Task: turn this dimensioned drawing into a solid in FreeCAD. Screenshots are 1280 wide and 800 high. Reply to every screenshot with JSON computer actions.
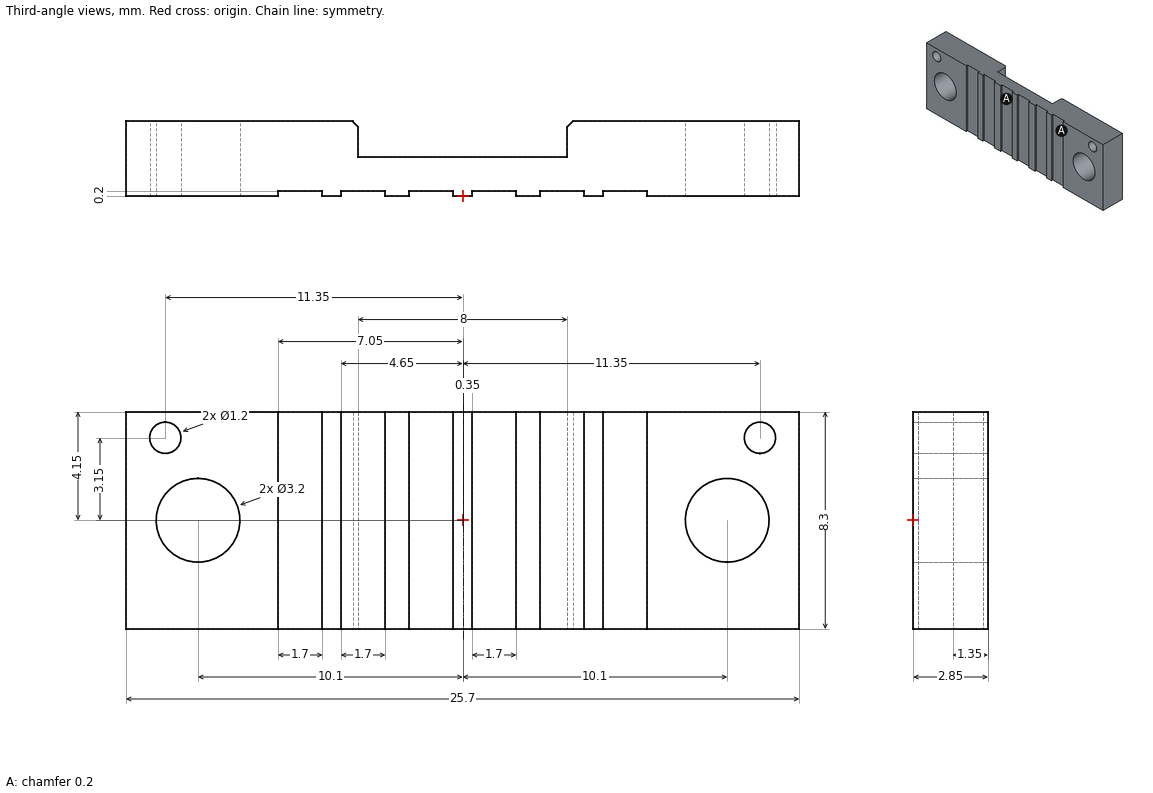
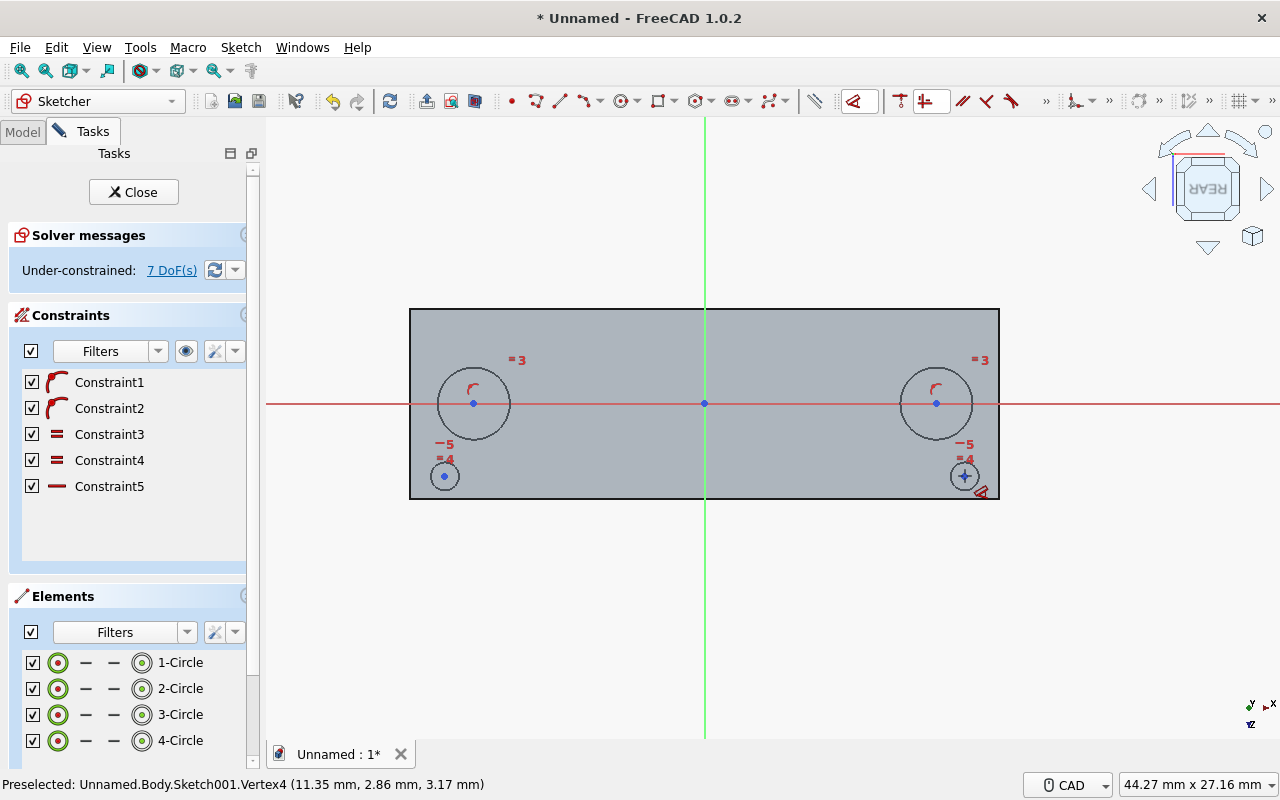
{"action": "left_click", "coordinate": [499, 378]}
{"action": "left_click", "coordinate": [521, 355]}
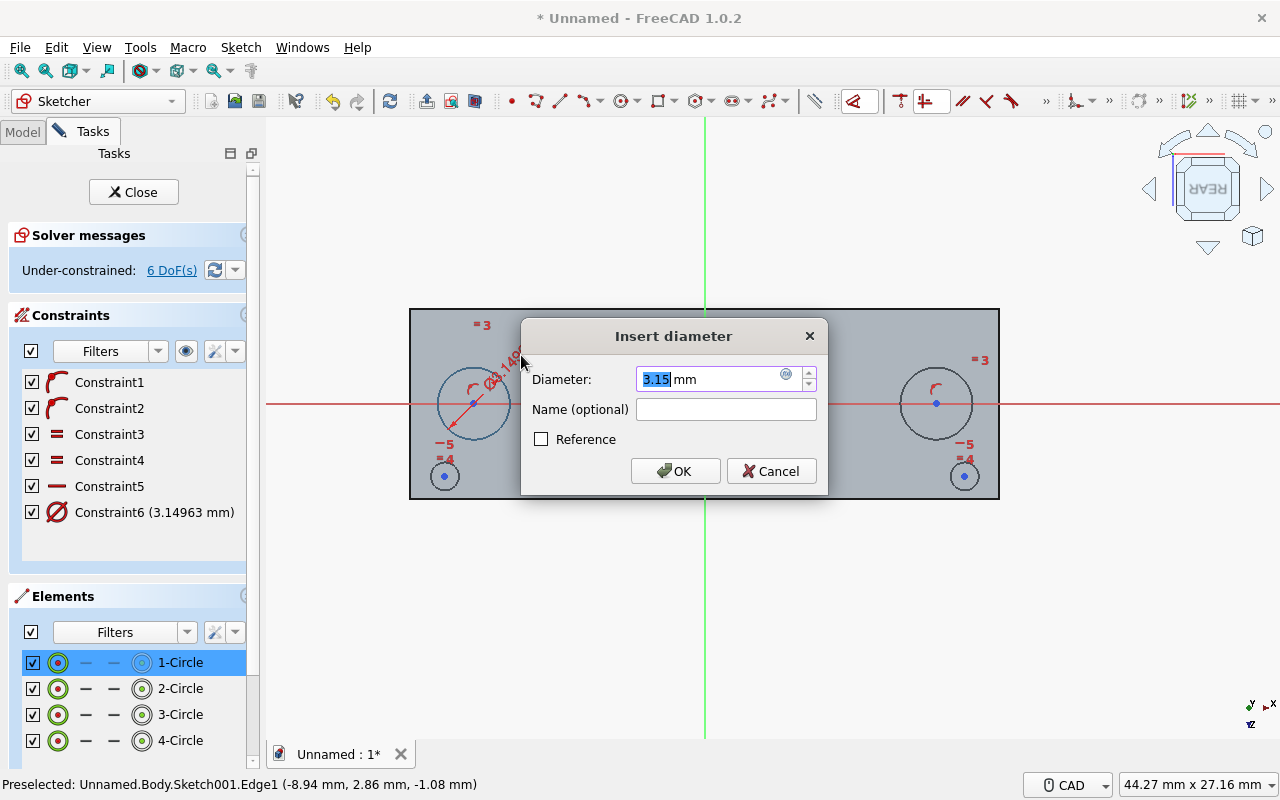
{"action": "type", "text": "3.2"}
{"action": "key", "text": "Return"}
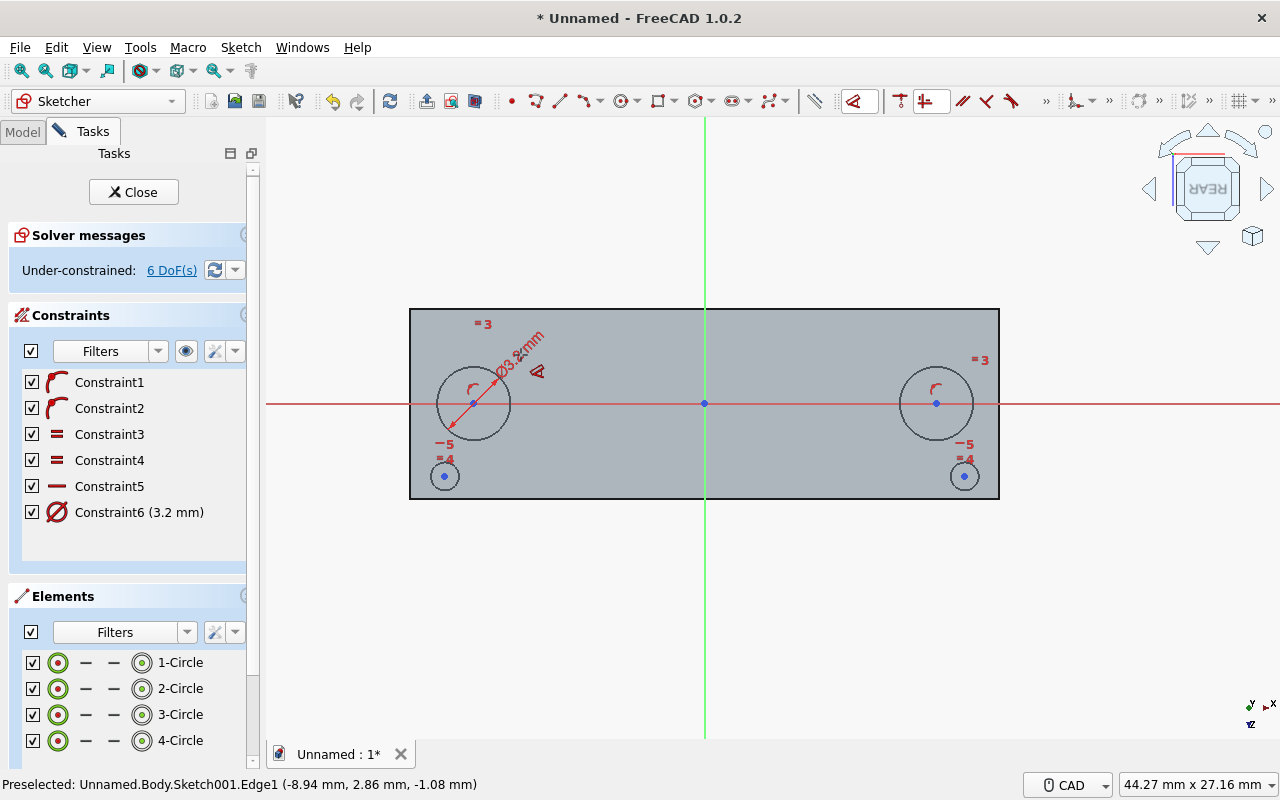
{"action": "scroll", "coordinate": [455, 467], "scroll_direction": "up", "scroll_amount": 2}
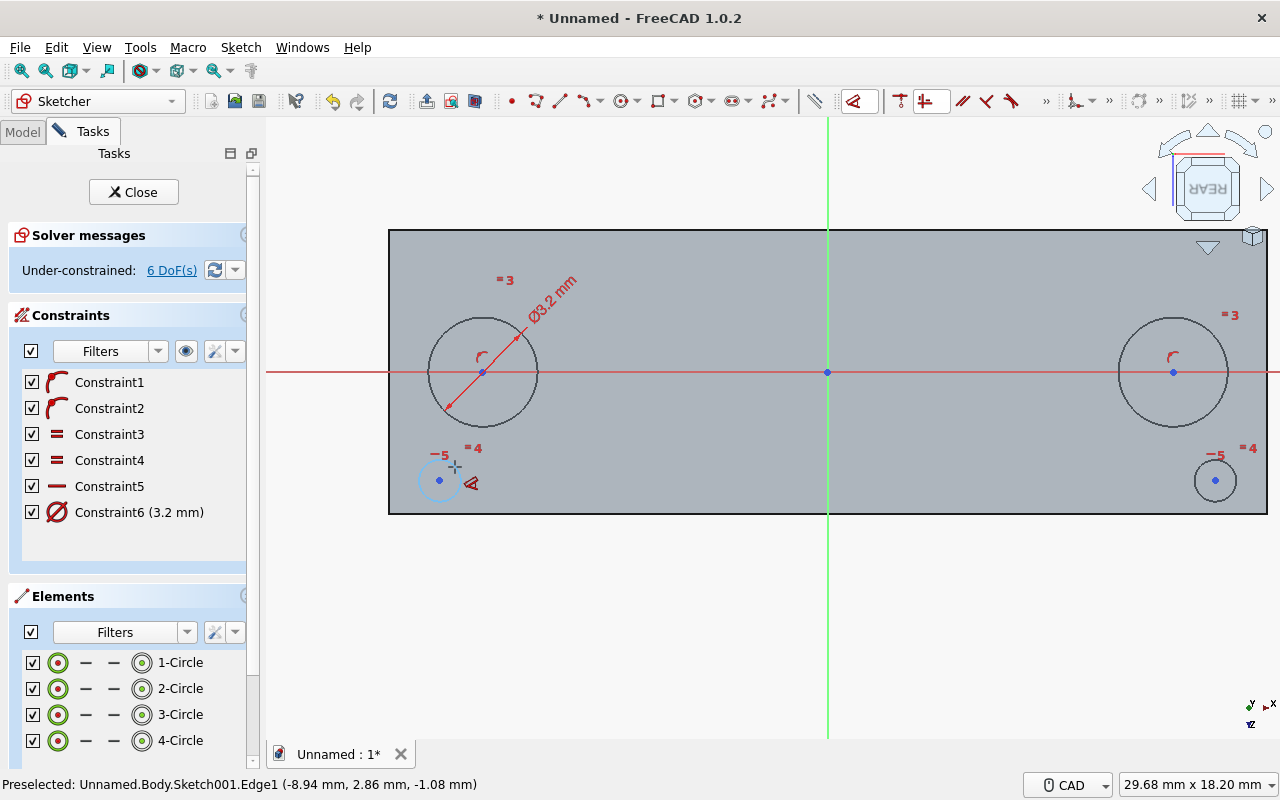
{"action": "left_click", "coordinate": [455, 466]}
{"action": "left_click", "coordinate": [478, 444]}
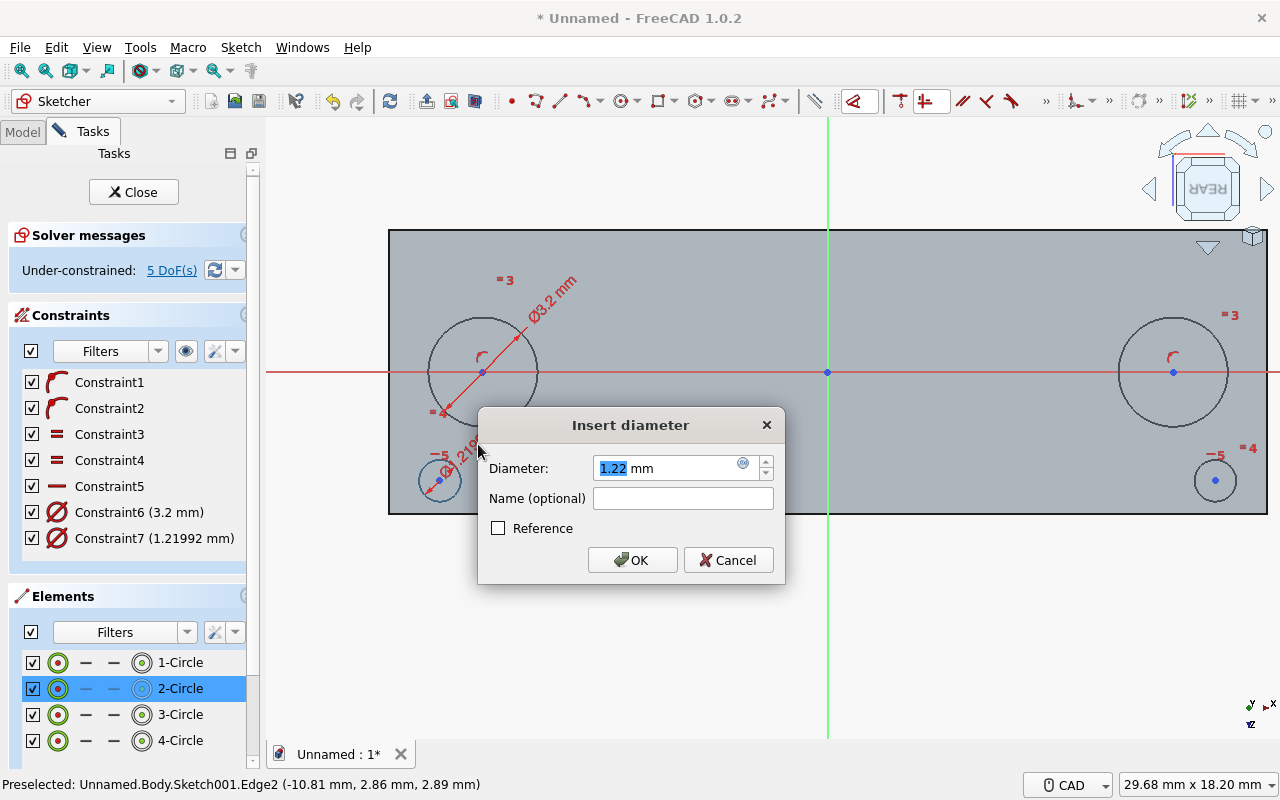
{"action": "type", "text": "1.2"}
{"action": "key", "text": "Return"}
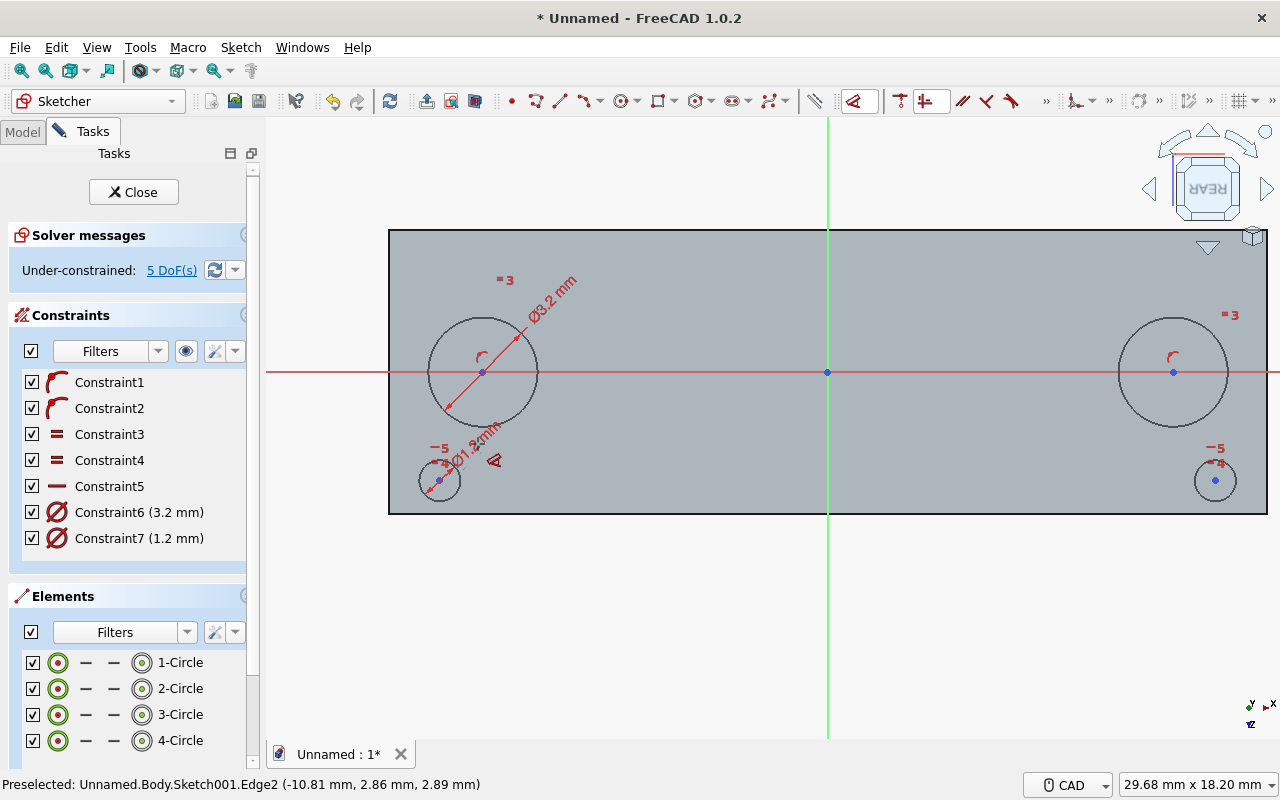
{"action": "left_click", "coordinate": [483, 372]}
{"action": "left_click", "coordinate": [655, 338]}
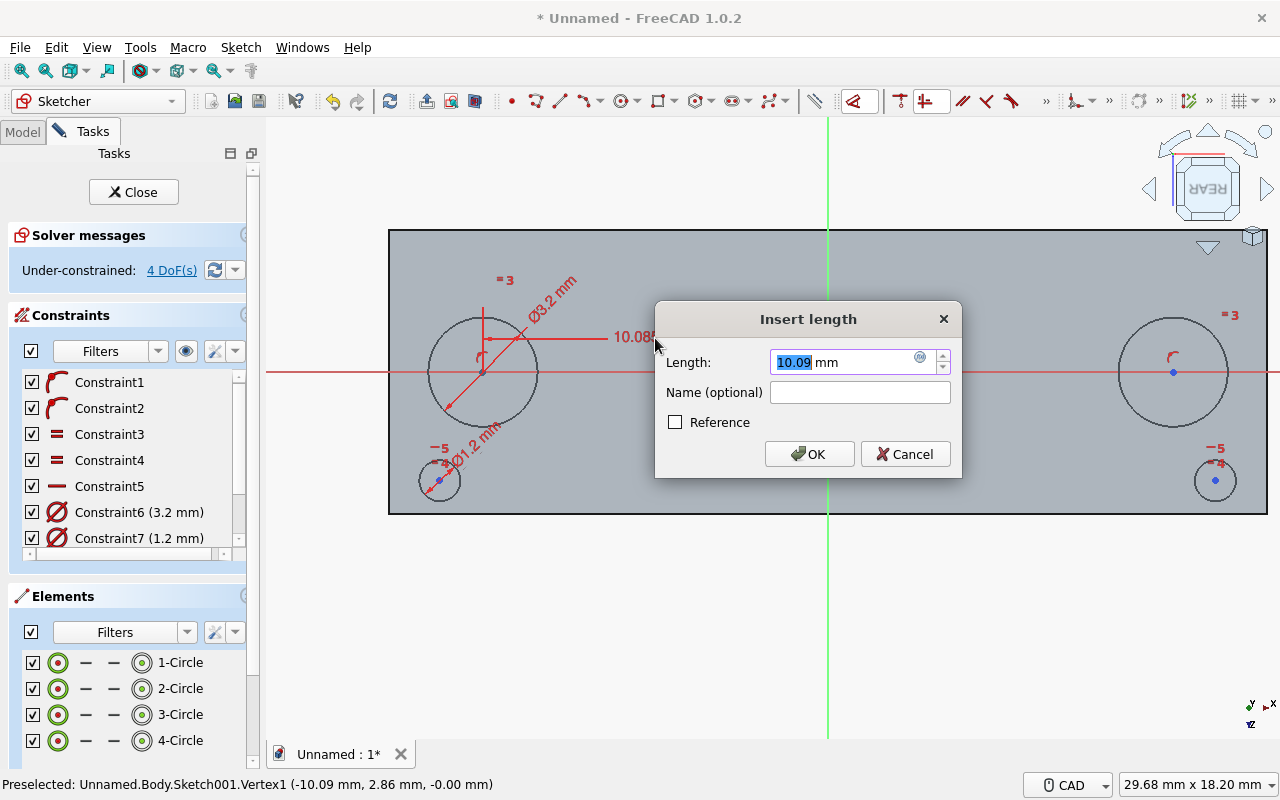
{"action": "type", "text": "10.1"}
{"action": "key", "text": "Return"}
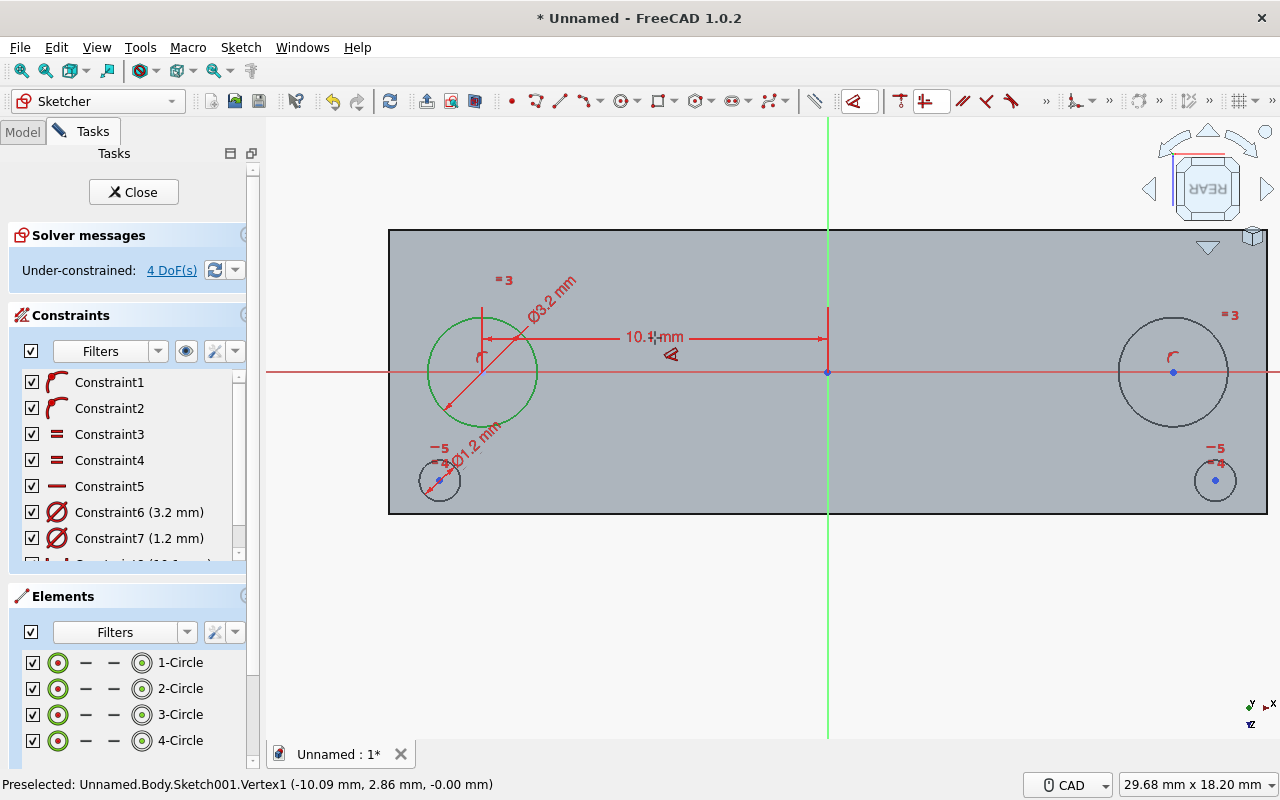
{"action": "left_click", "coordinate": [440, 481]}
{"action": "left_click", "coordinate": [406, 426]}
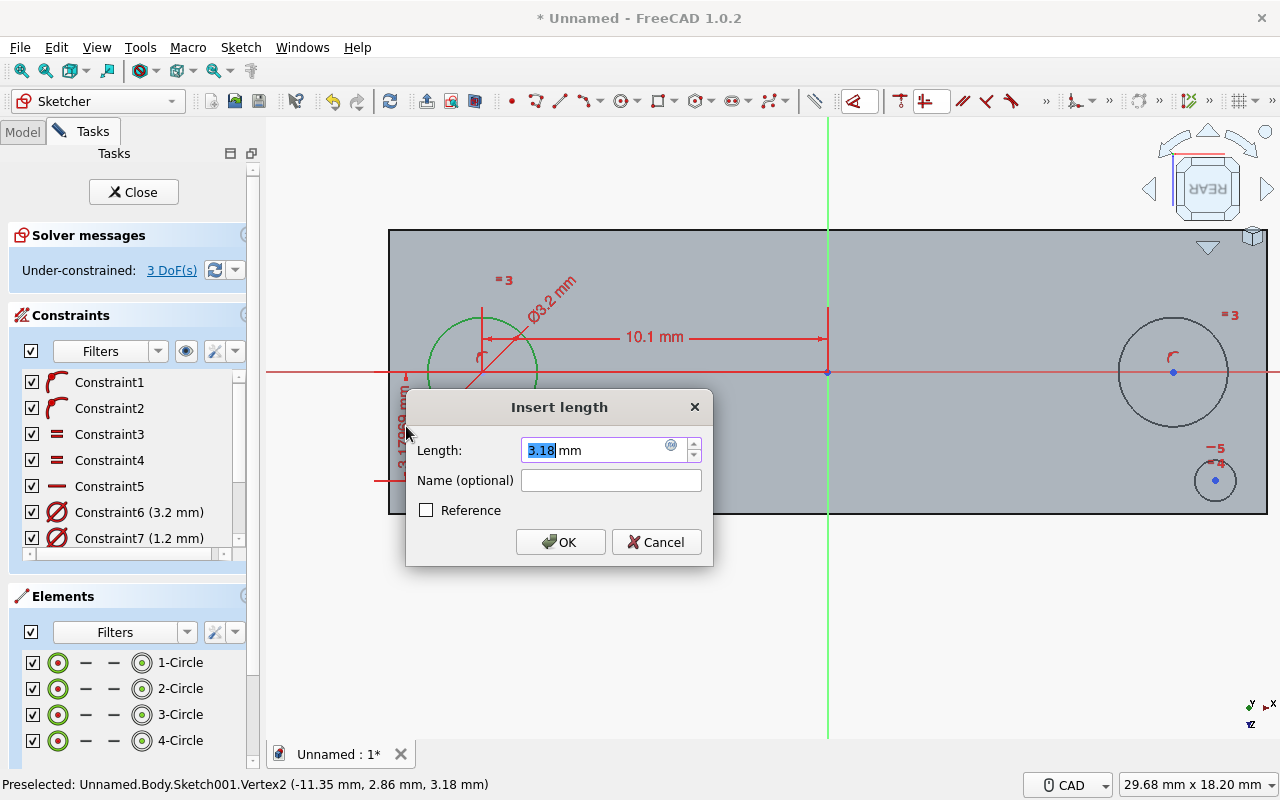
{"action": "type", "text": "3.15"}
{"action": "key", "text": "Return"}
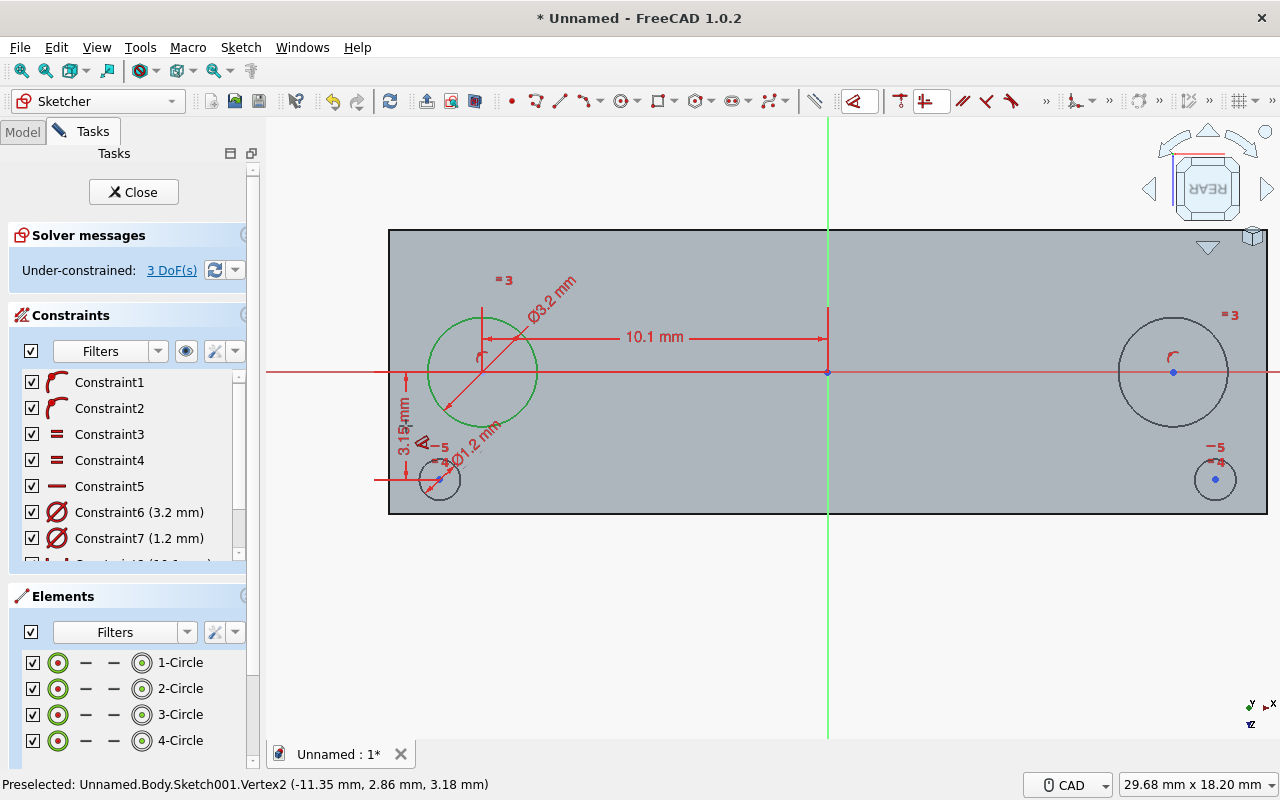
{"action": "scroll", "coordinate": [454, 467], "scroll_direction": "down", "scroll_amount": 2}